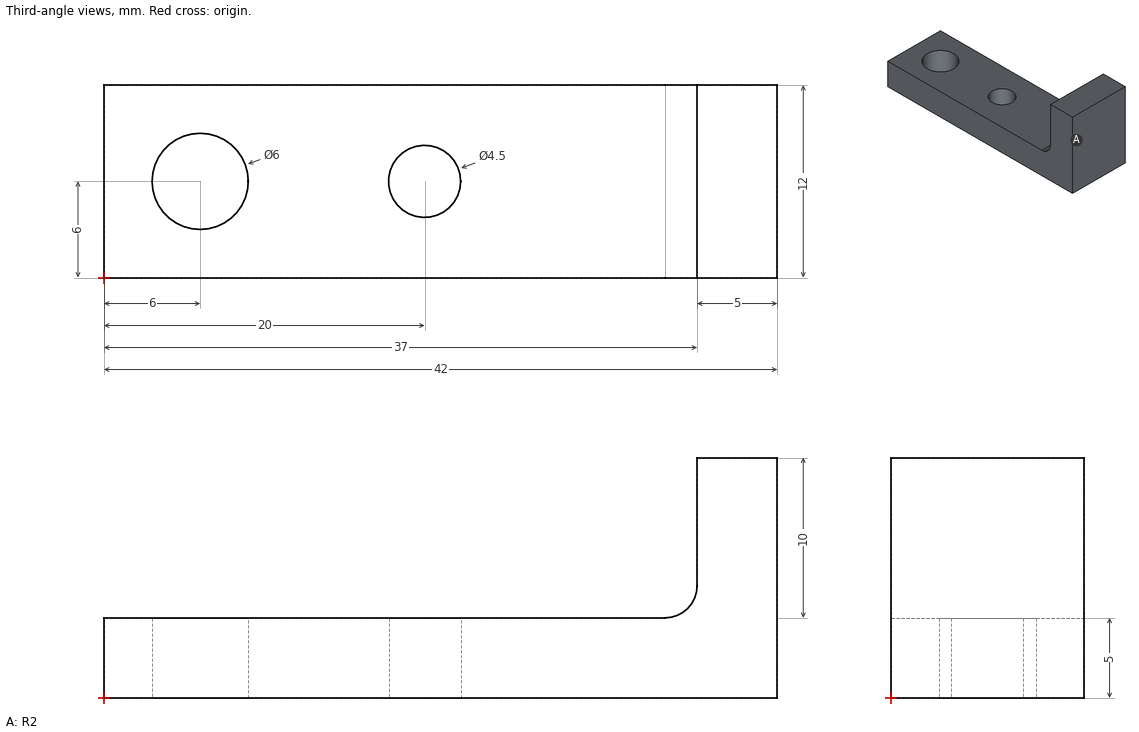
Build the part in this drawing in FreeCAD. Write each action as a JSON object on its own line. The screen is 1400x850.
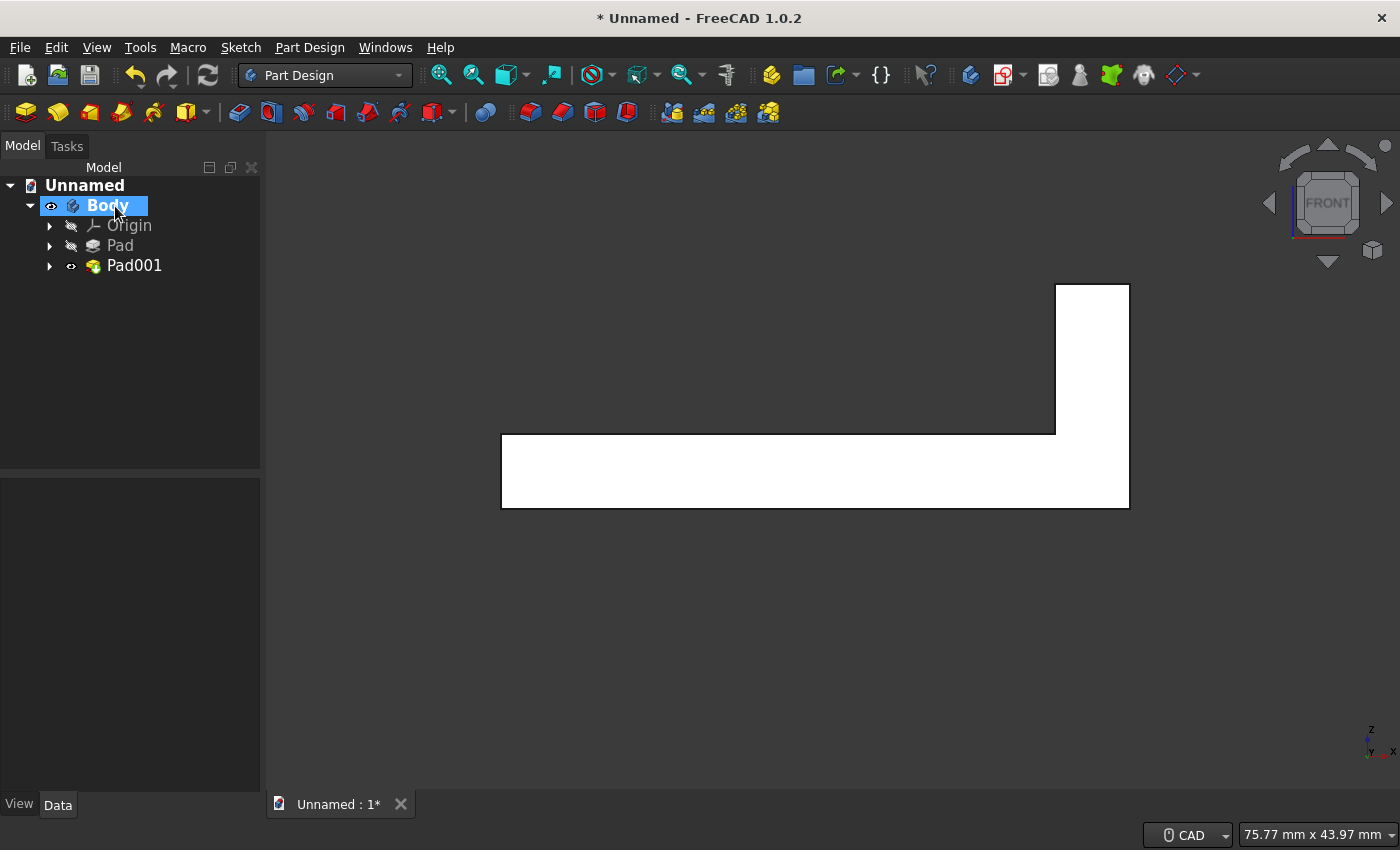
{"action": "key", "text": "3"}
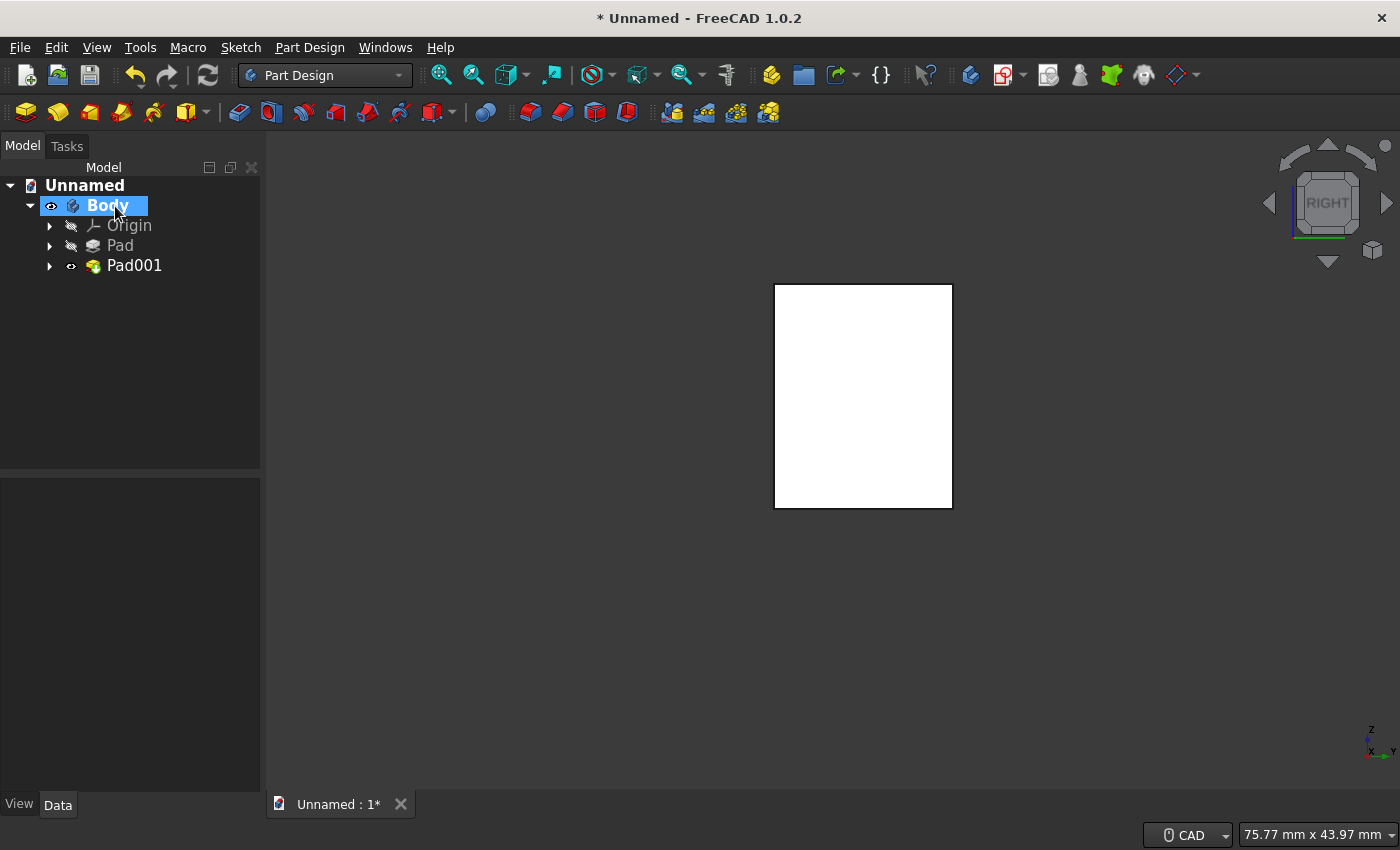
{"action": "key", "text": "v f"}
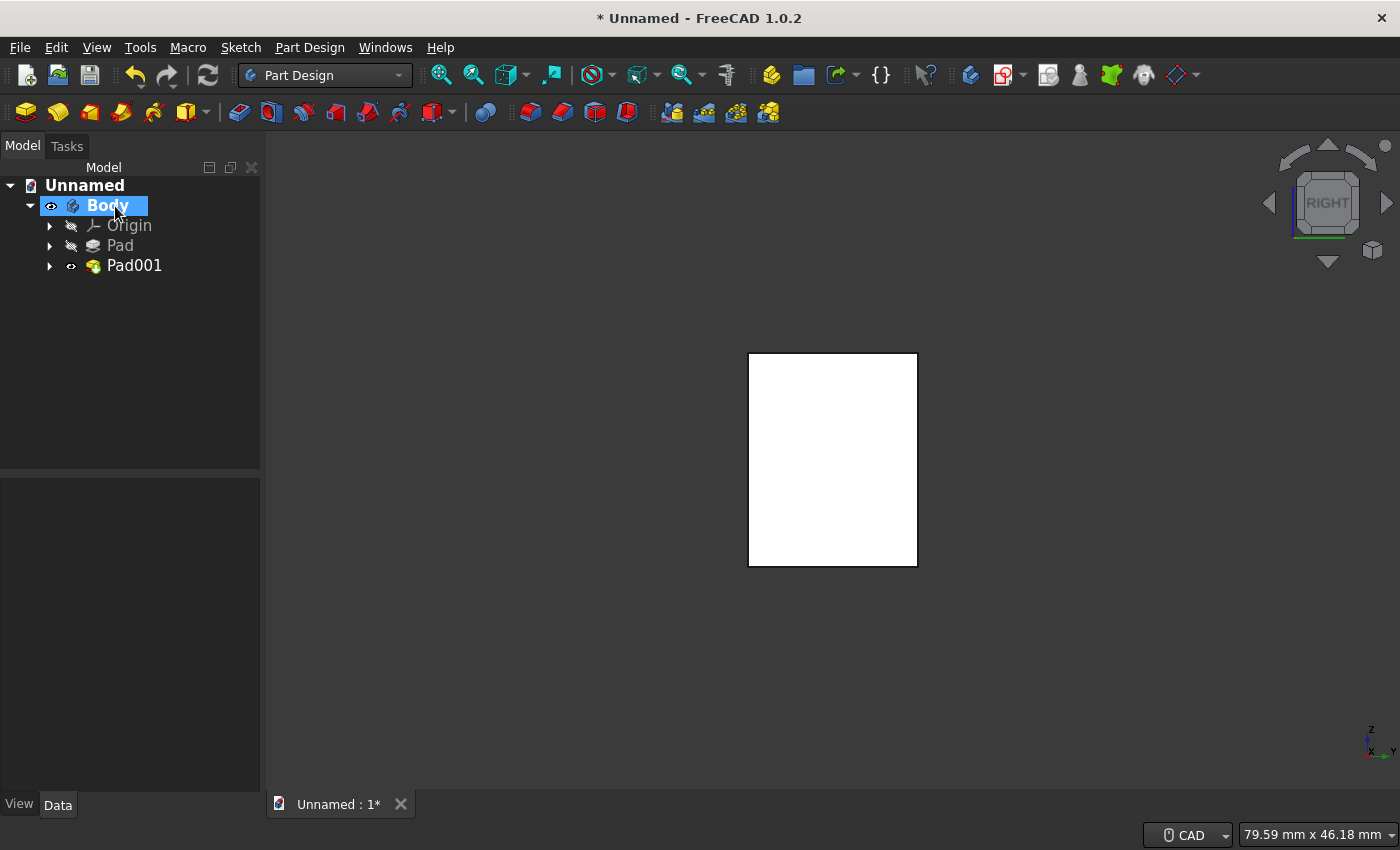
{"action": "key", "text": "5"}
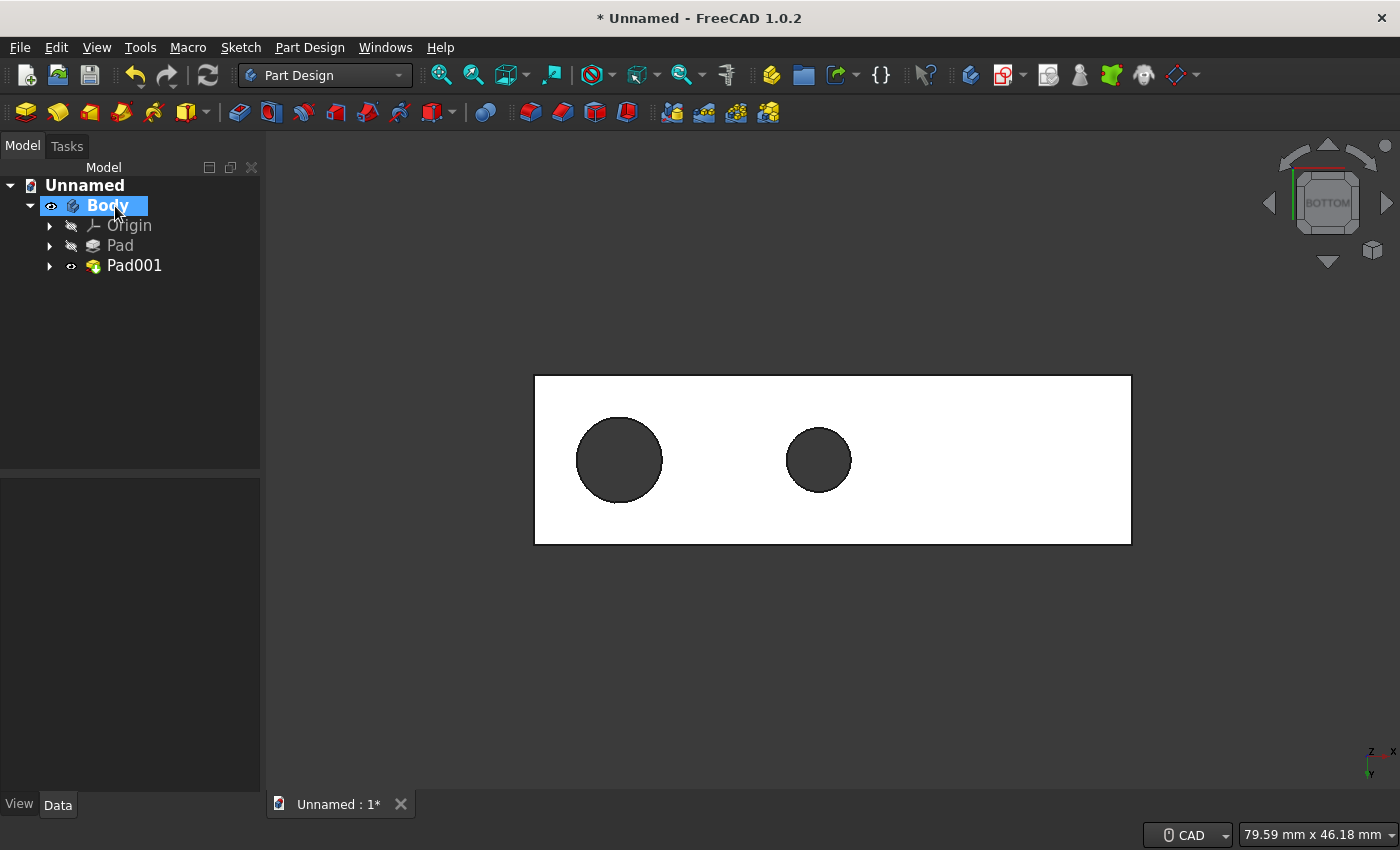
{"action": "key", "text": "4"}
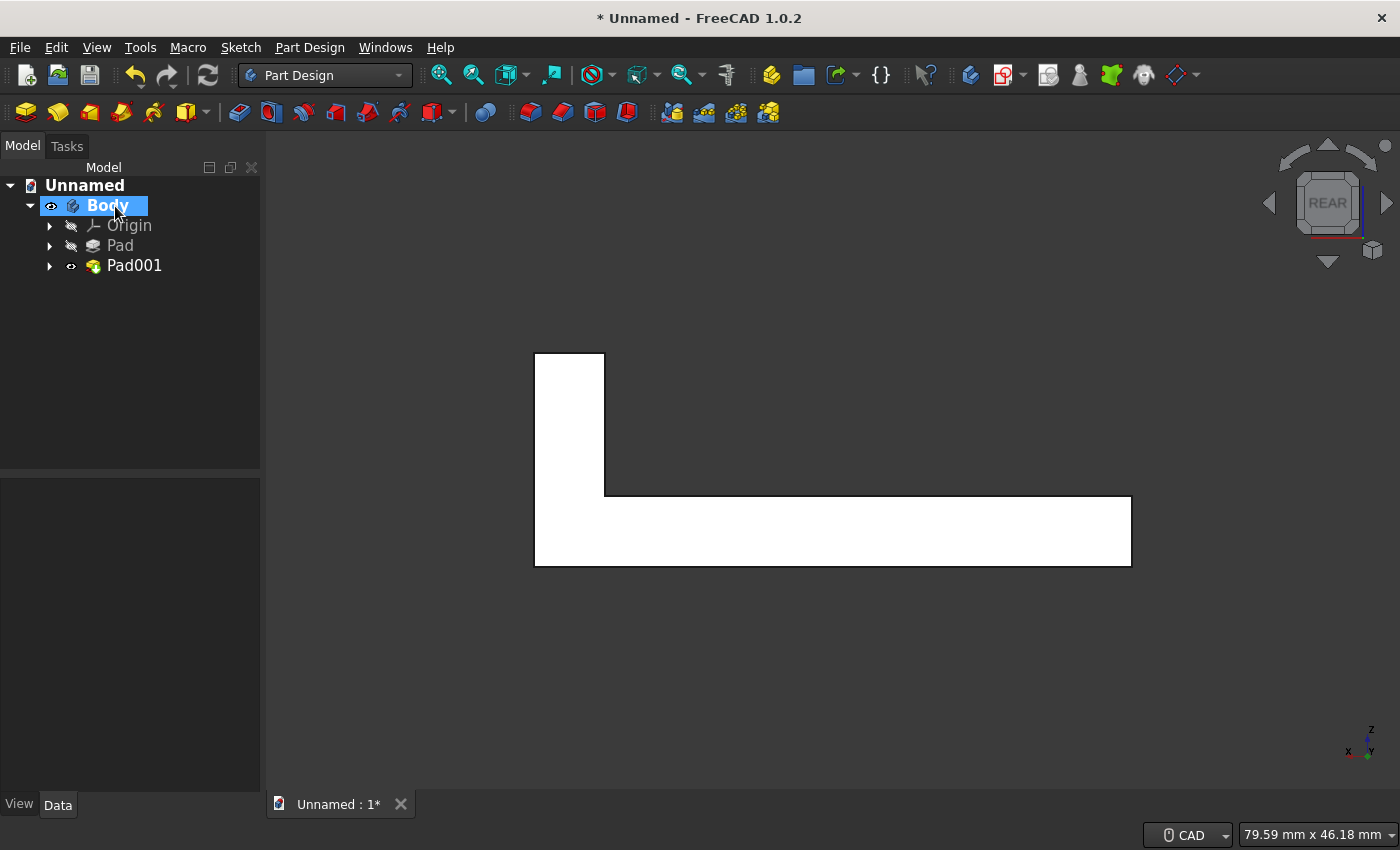
{"action": "key", "text": "6"}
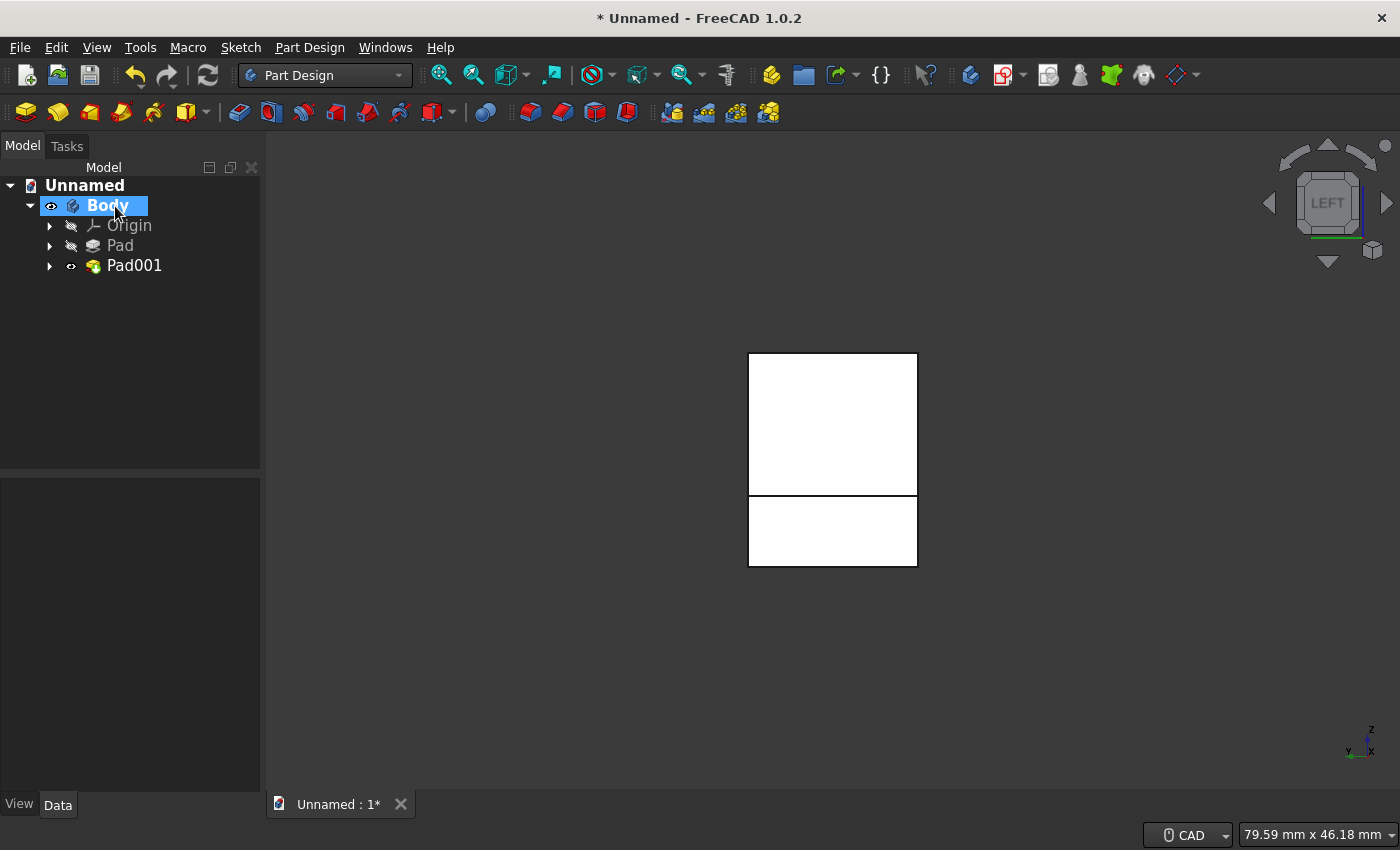
{"action": "left_click", "coordinate": [442, 76]}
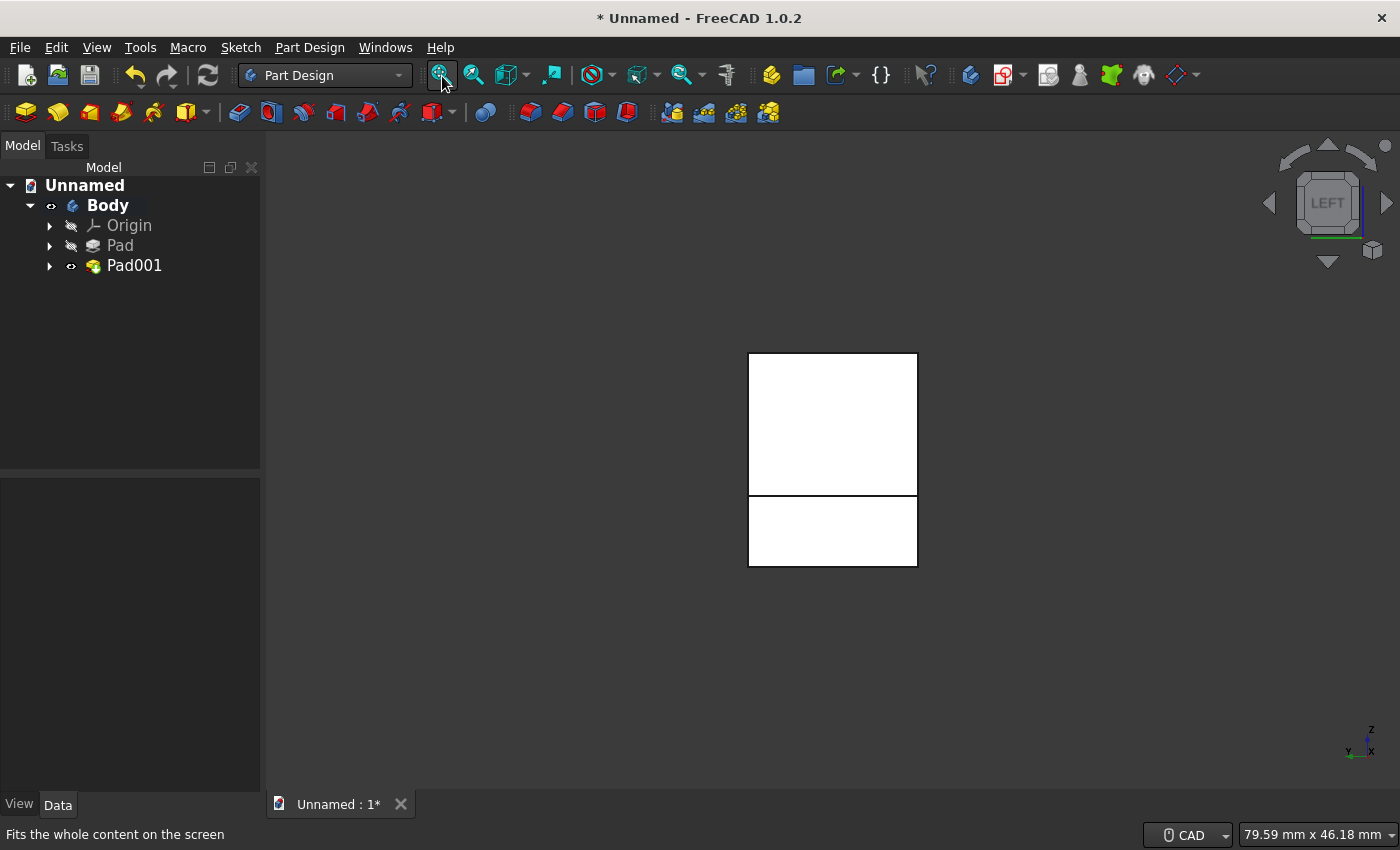
{"action": "key", "text": "v 3"}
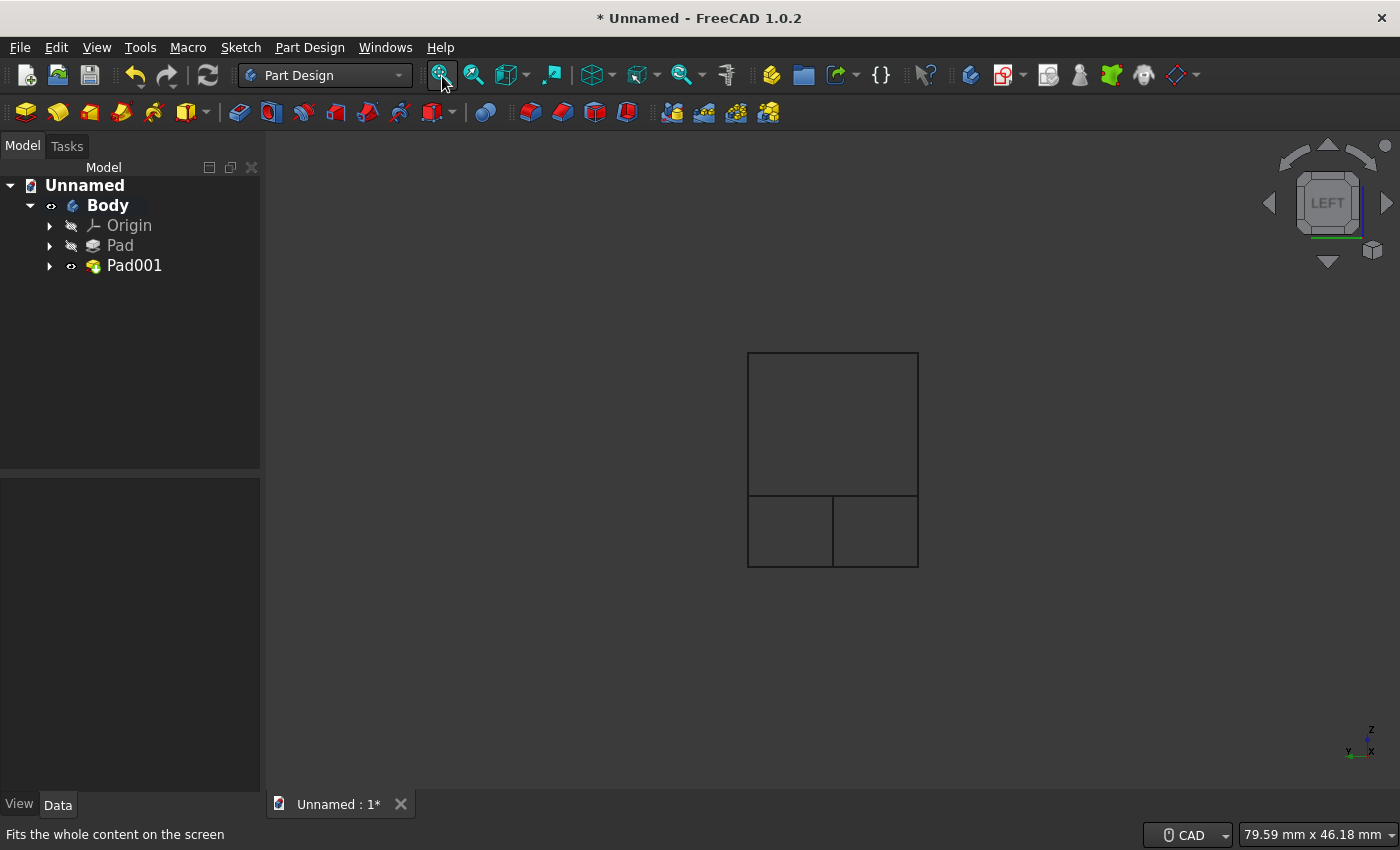
{"action": "key", "text": "0"}